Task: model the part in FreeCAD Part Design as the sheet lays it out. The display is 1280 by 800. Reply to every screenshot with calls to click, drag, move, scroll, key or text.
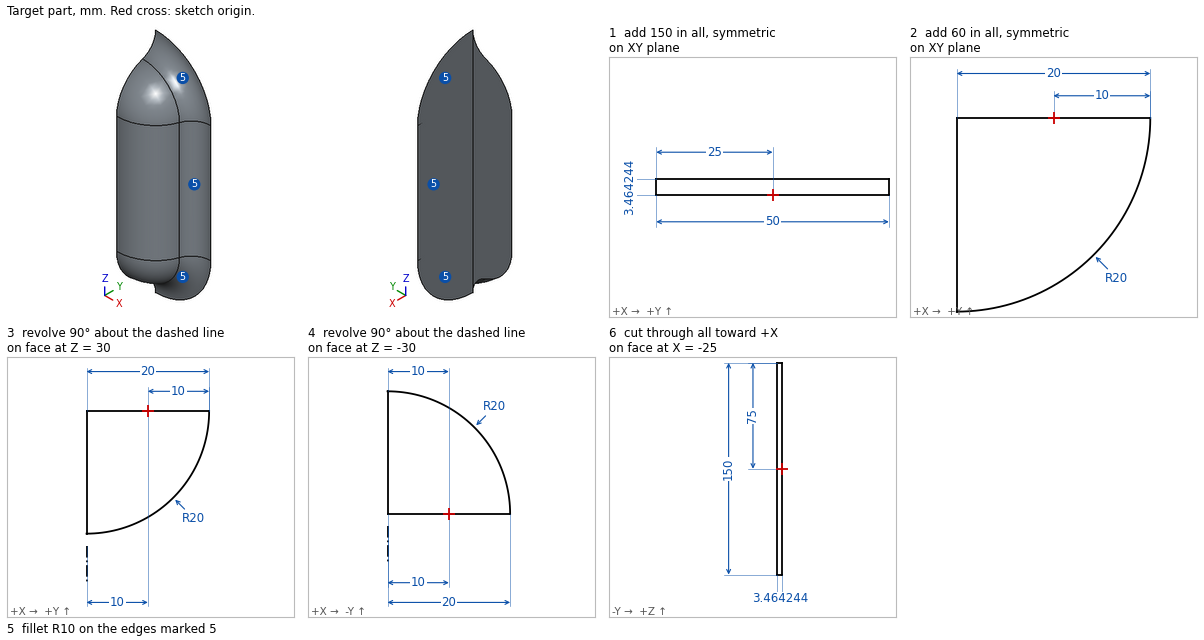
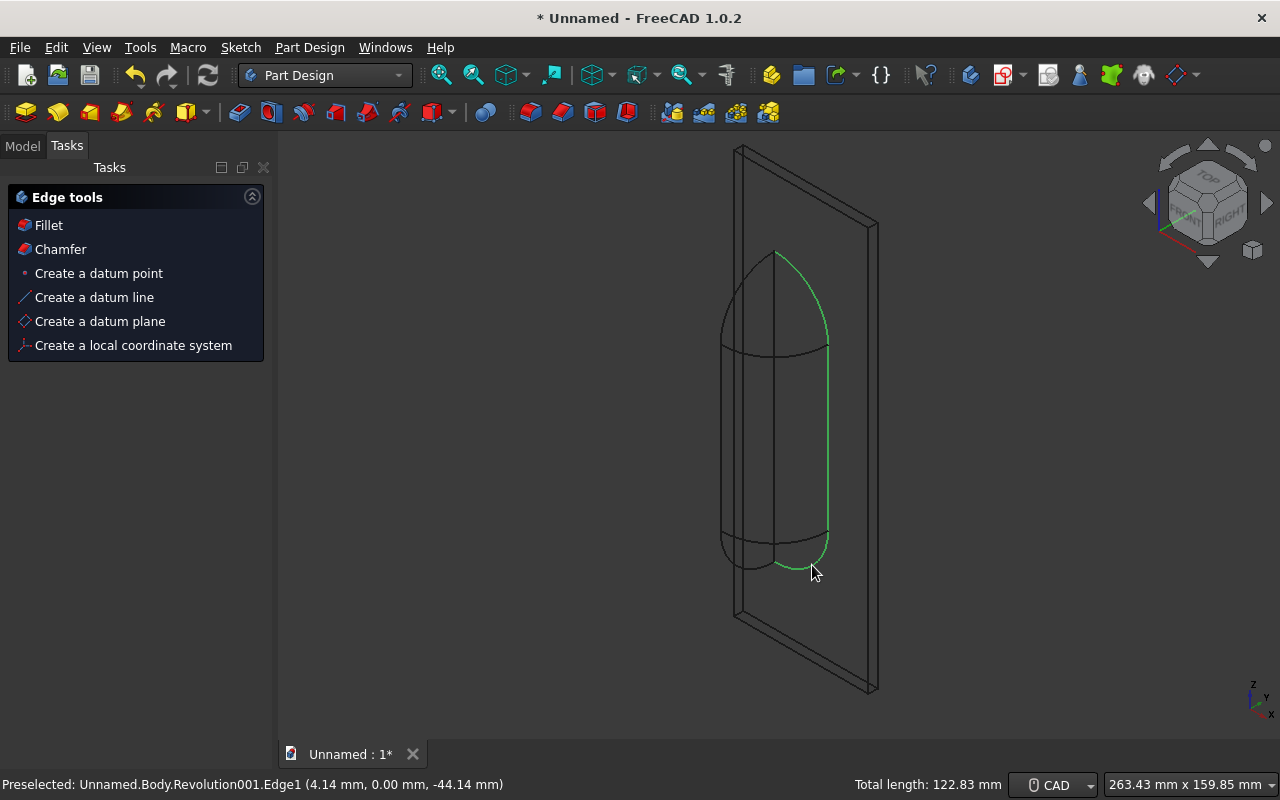
key(v)
key(1)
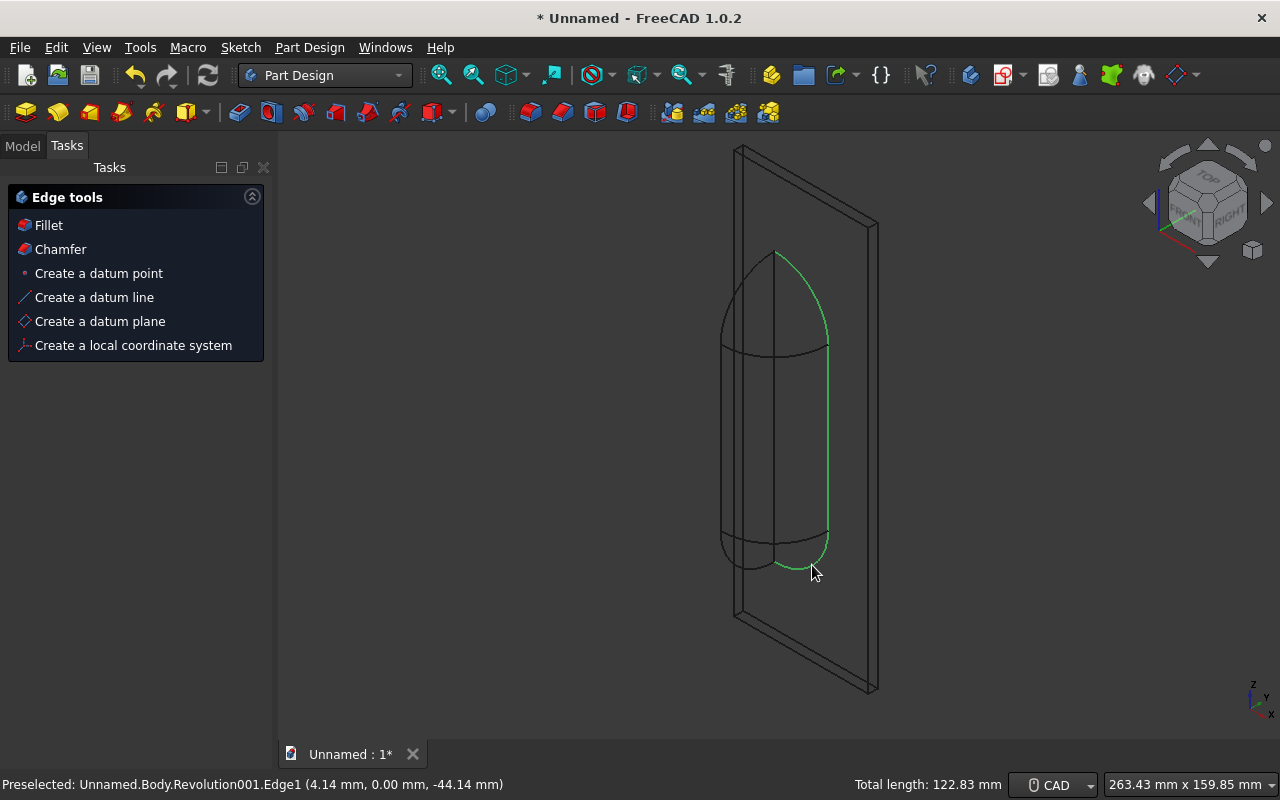
click(532, 112)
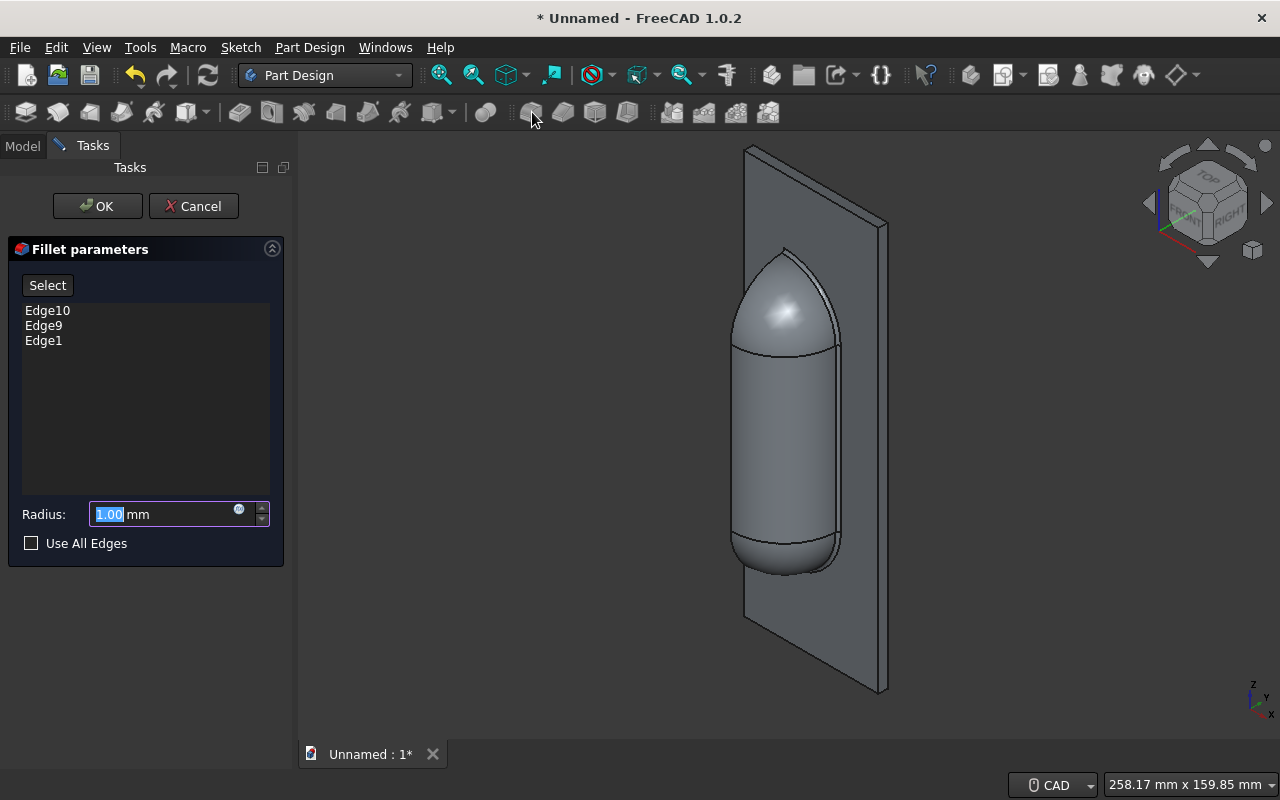
text(10)
key(Tab)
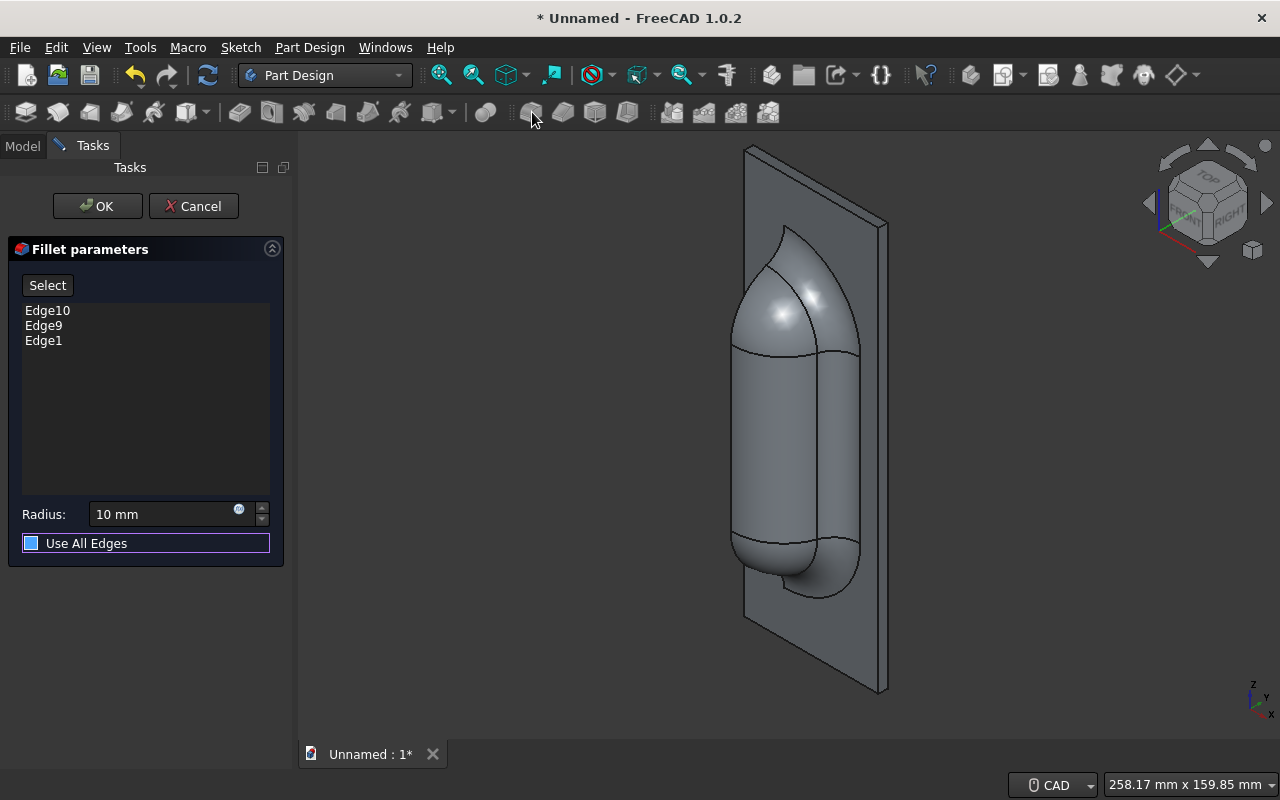
click(98, 206)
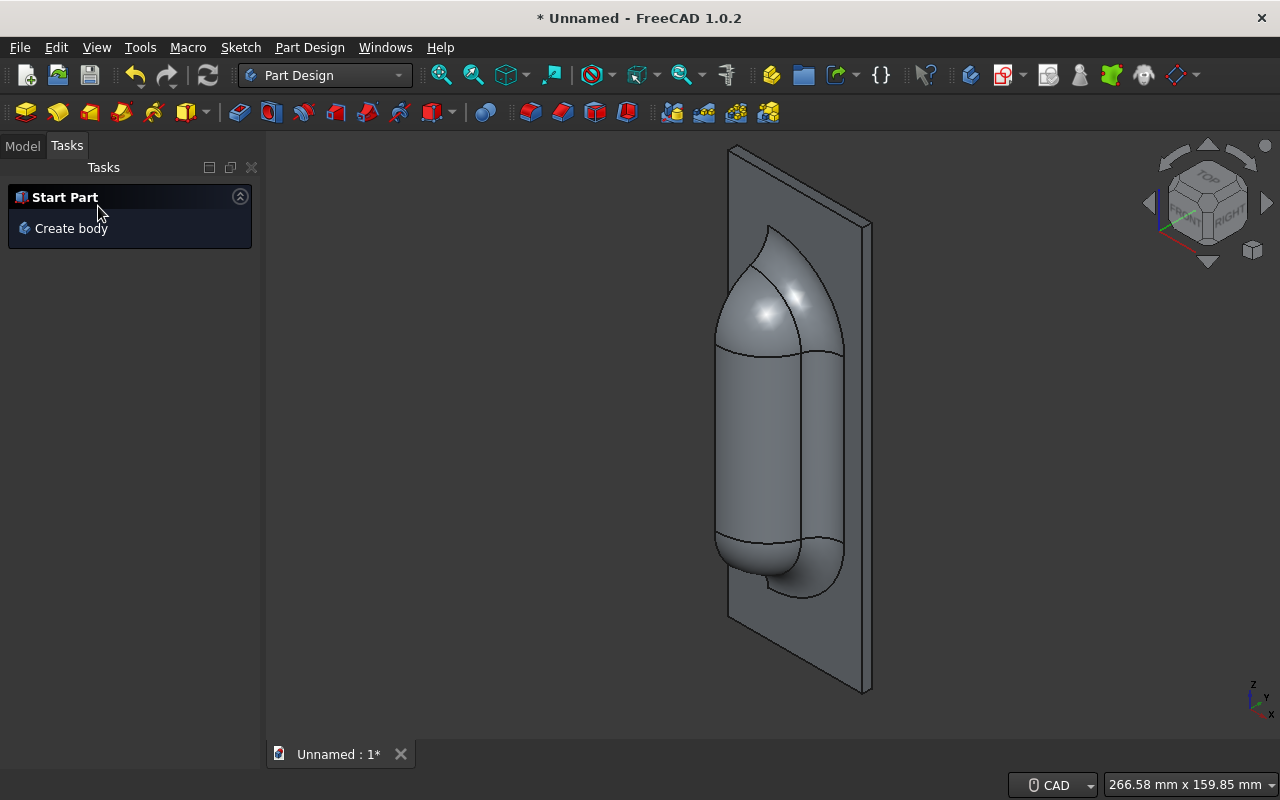
key(6)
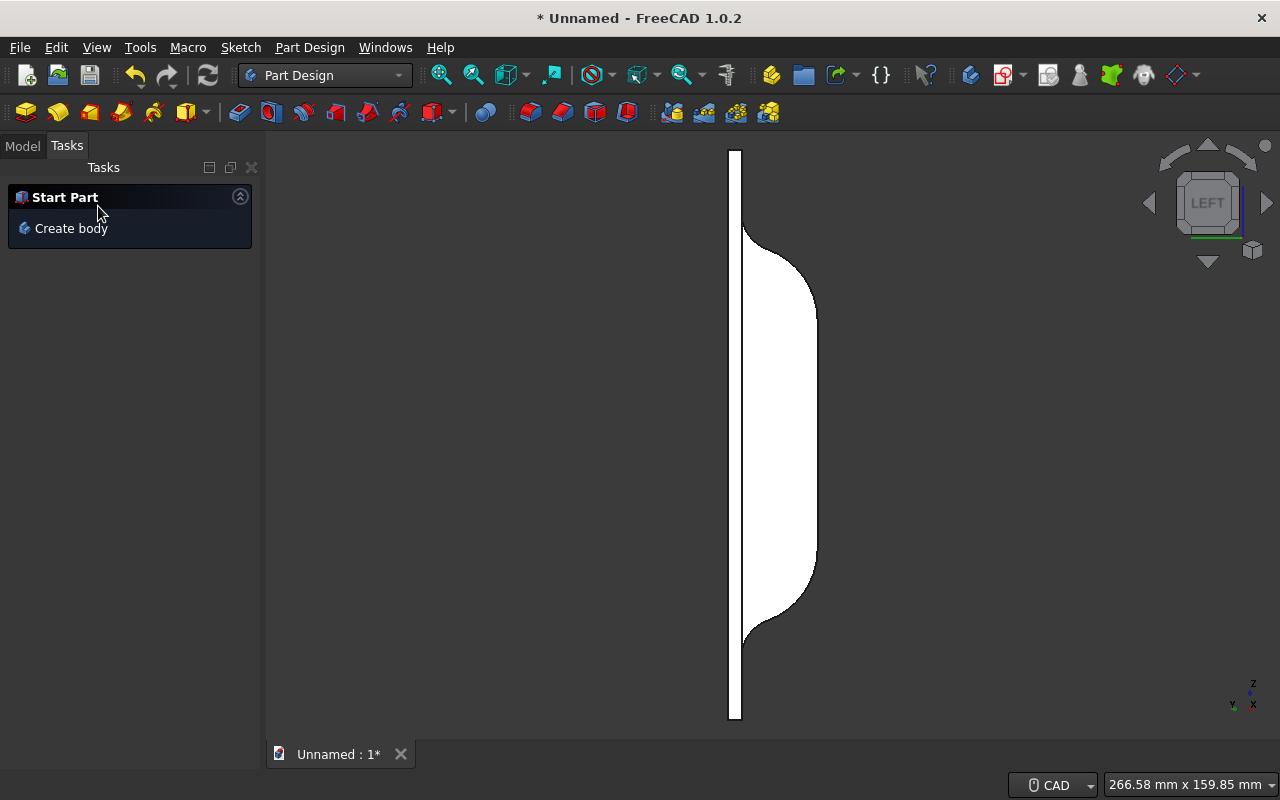
scroll(735, 189, up, 3)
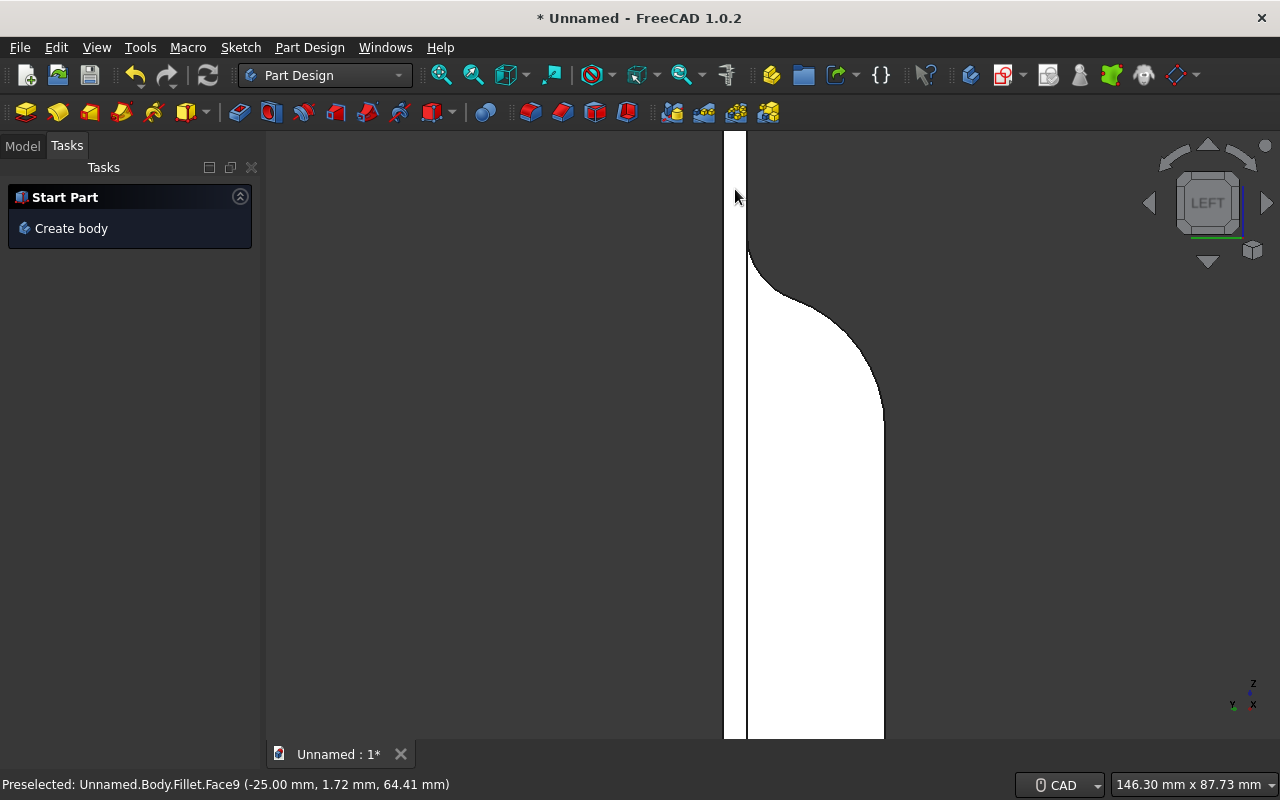
click(735, 191)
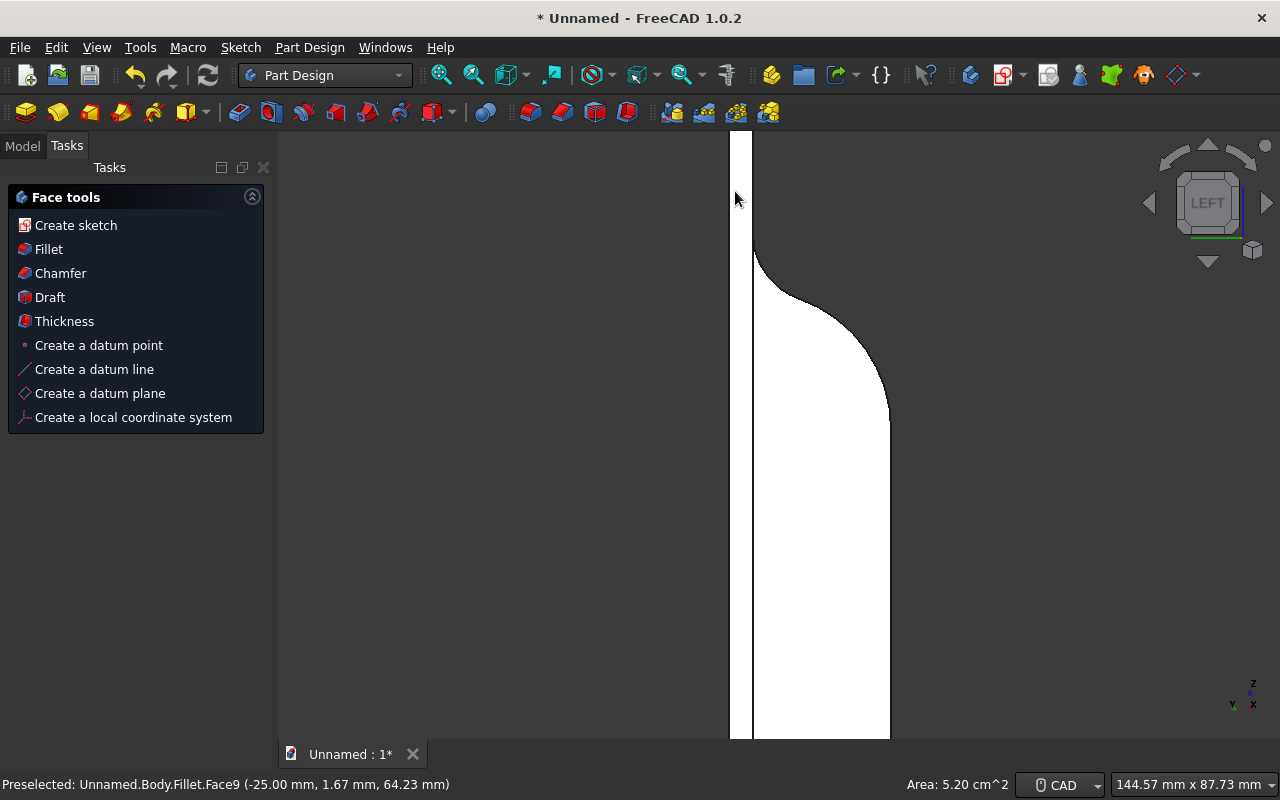
click(1004, 76)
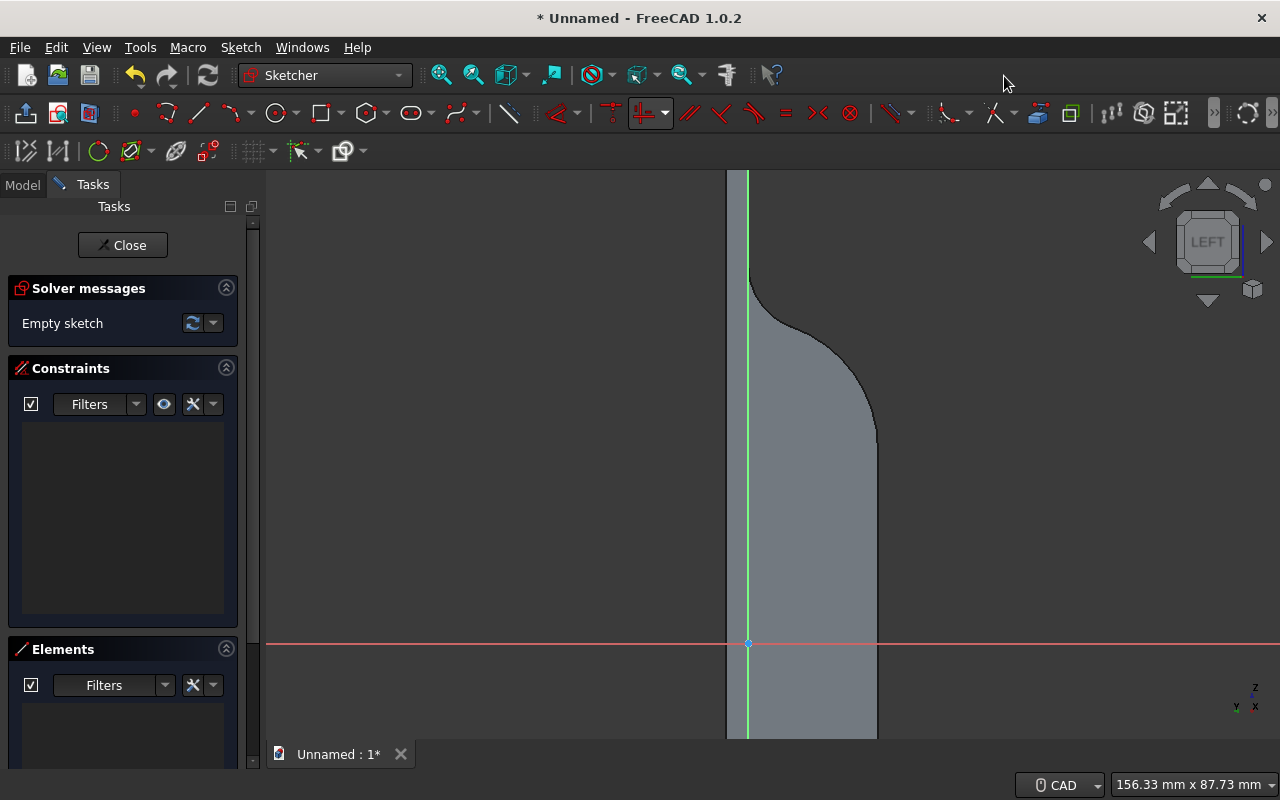
scroll(686, 344, down, 5)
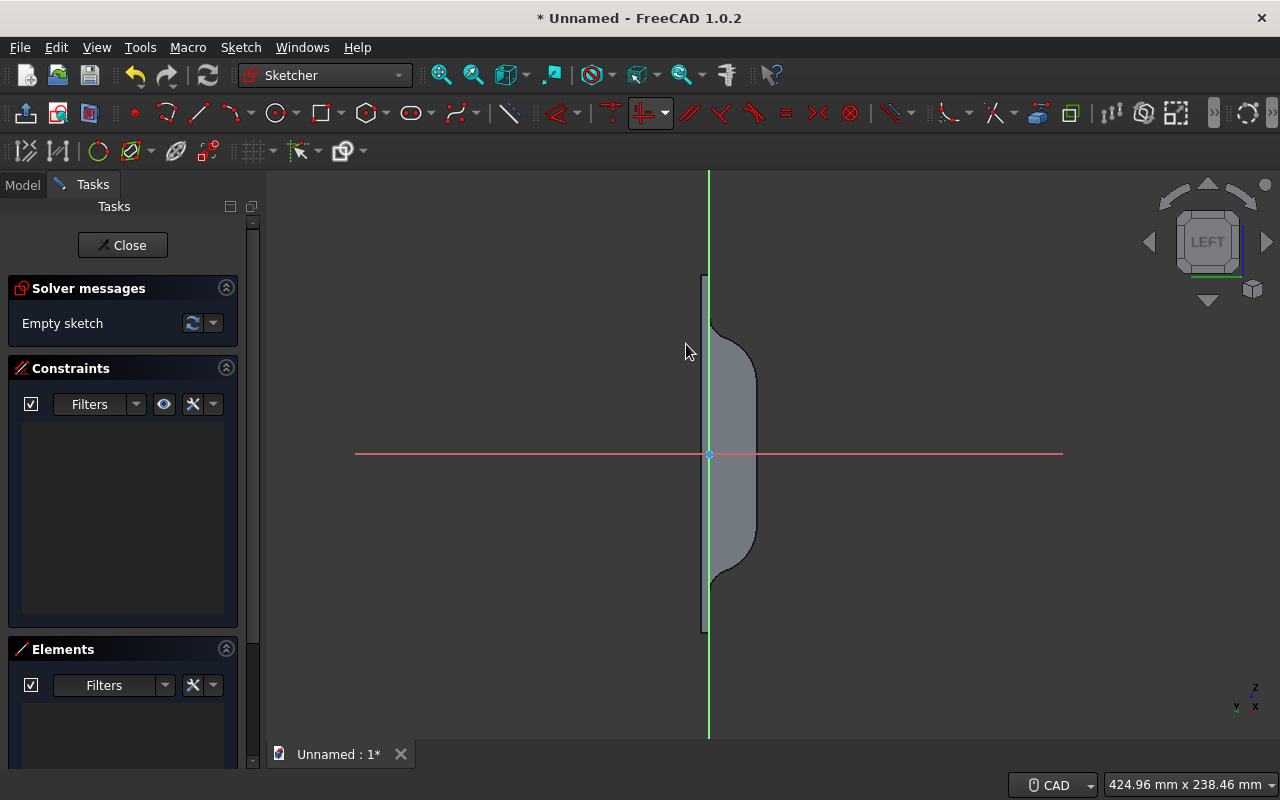
click(322, 114)